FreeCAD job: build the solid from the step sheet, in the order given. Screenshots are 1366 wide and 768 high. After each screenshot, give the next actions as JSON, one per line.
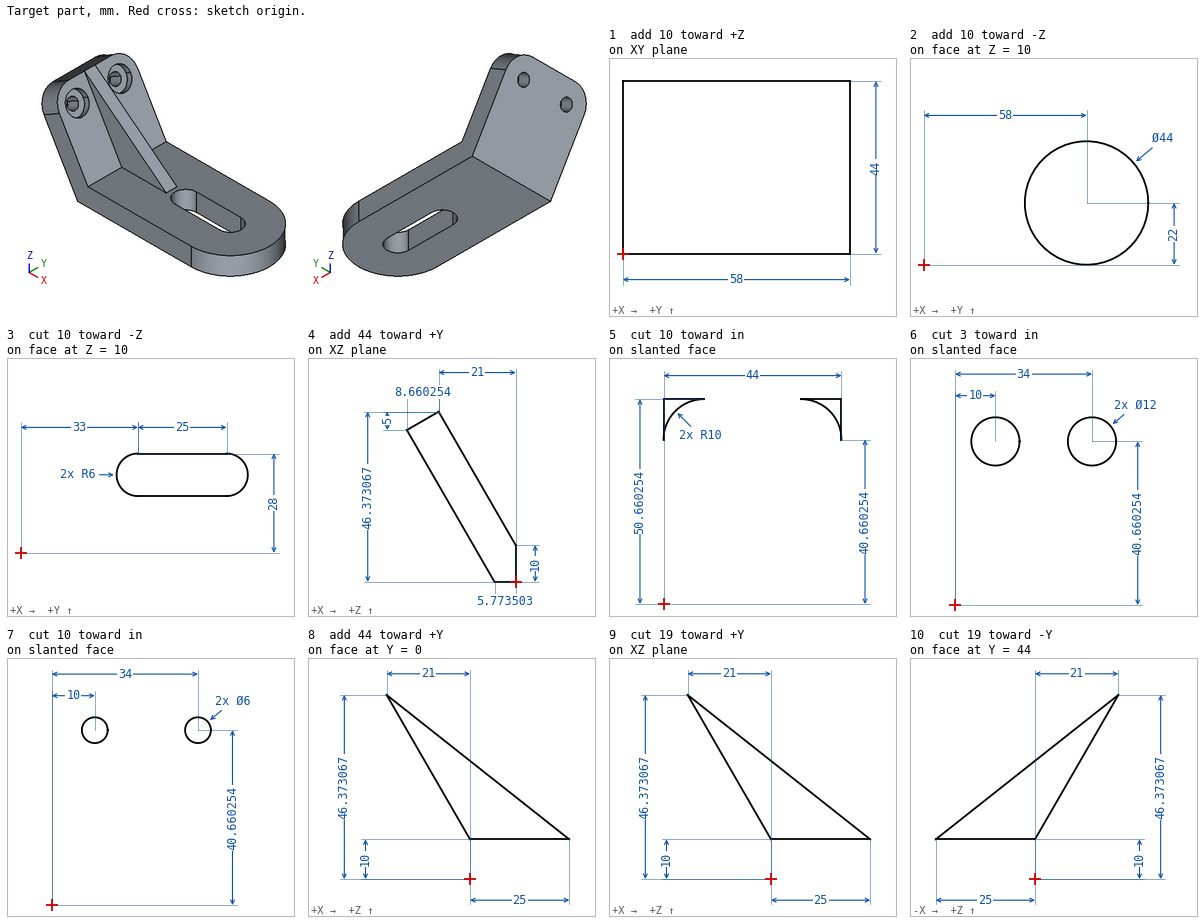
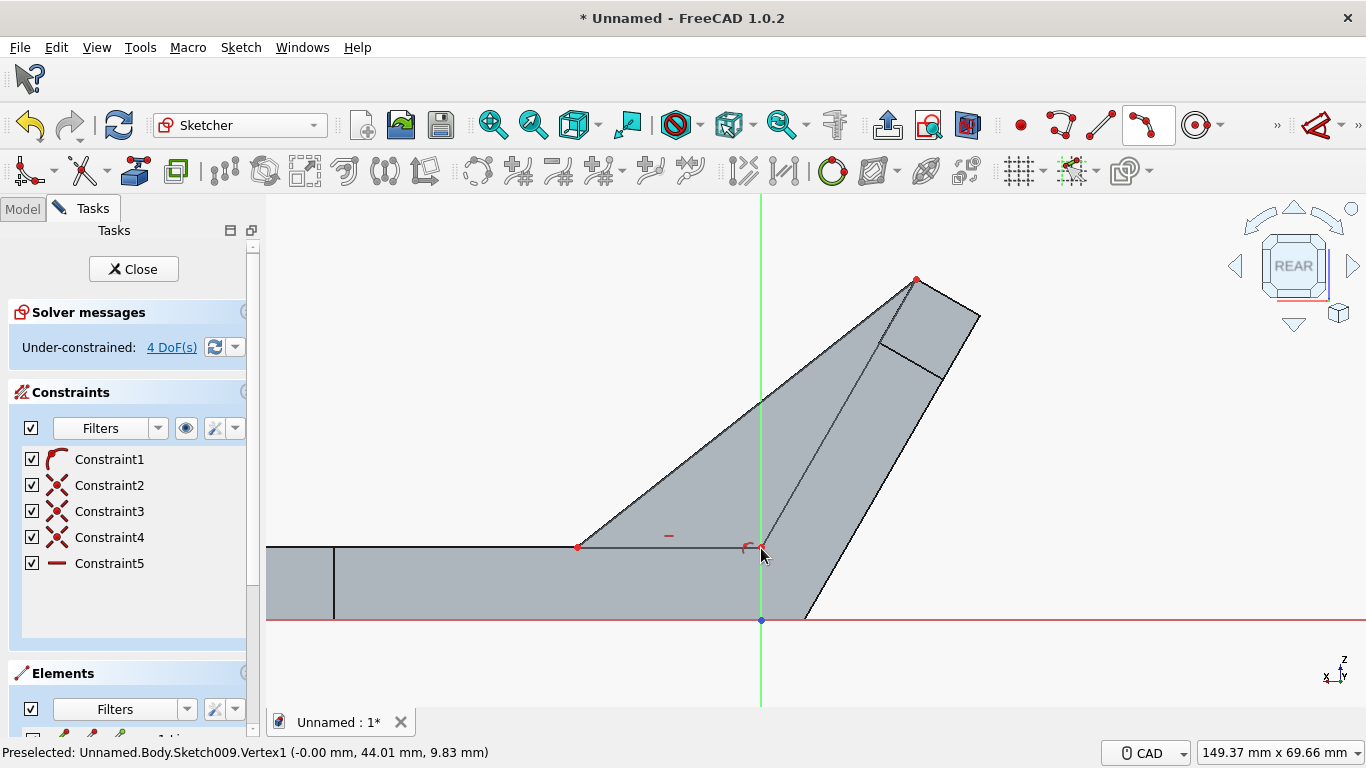
{"action": "left_click", "coordinate": [1316, 126]}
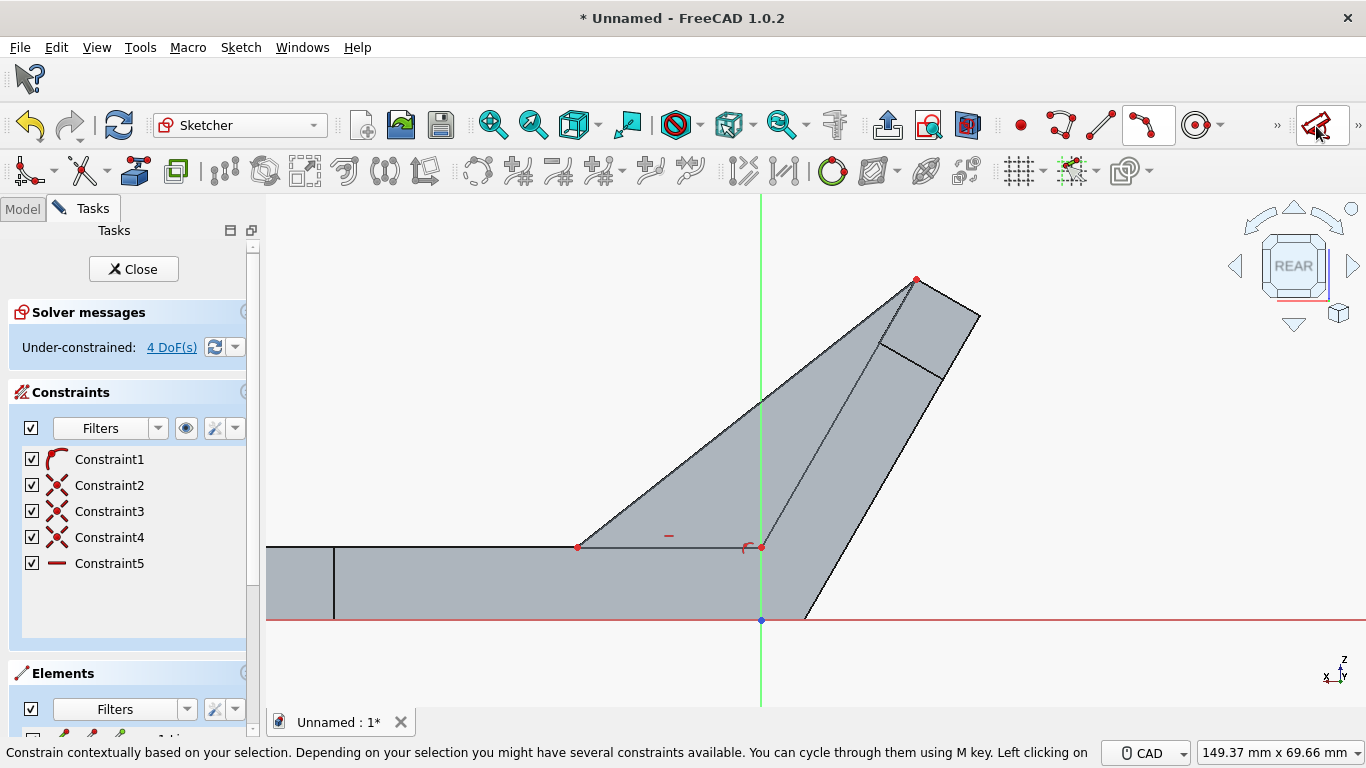
{"action": "left_click", "coordinate": [632, 548]}
{"action": "left_click", "coordinate": [669, 582]}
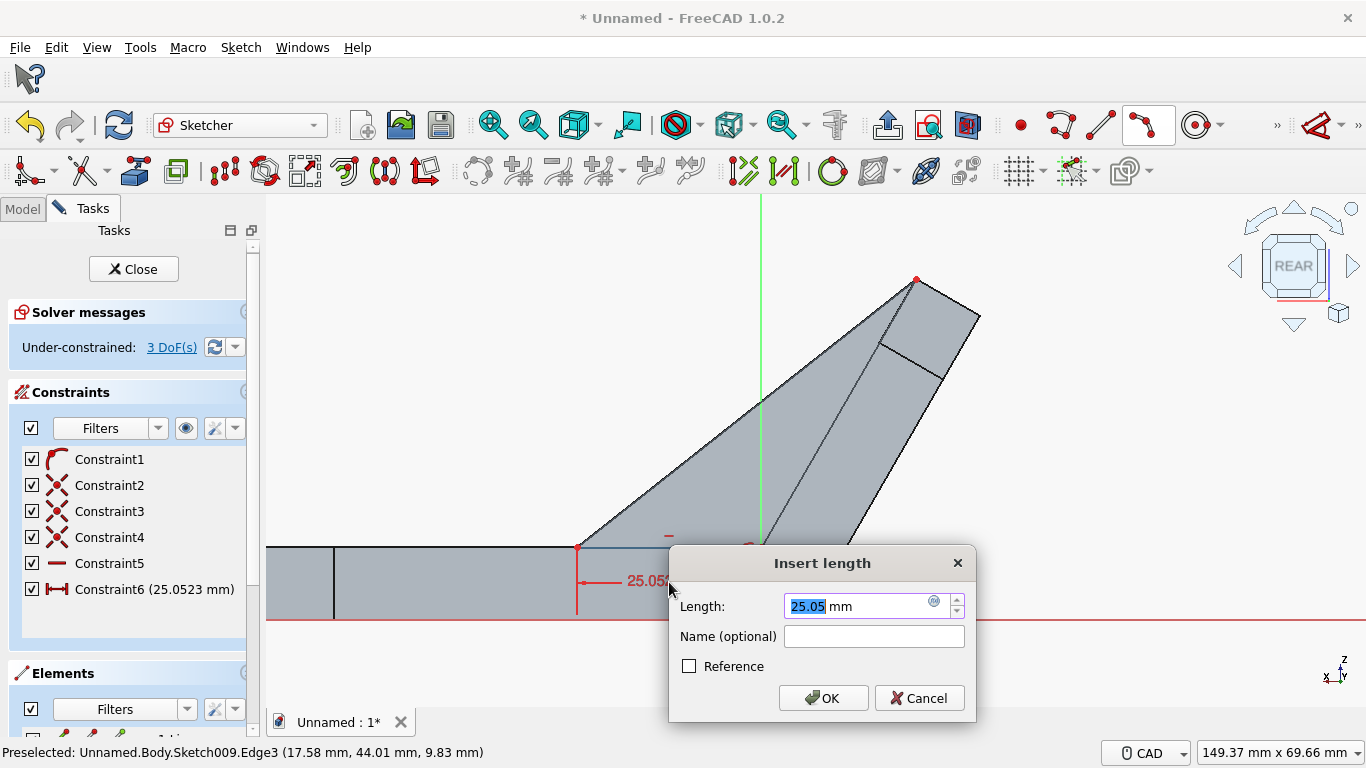
{"action": "type", "text": "25"}
{"action": "key", "text": "Return"}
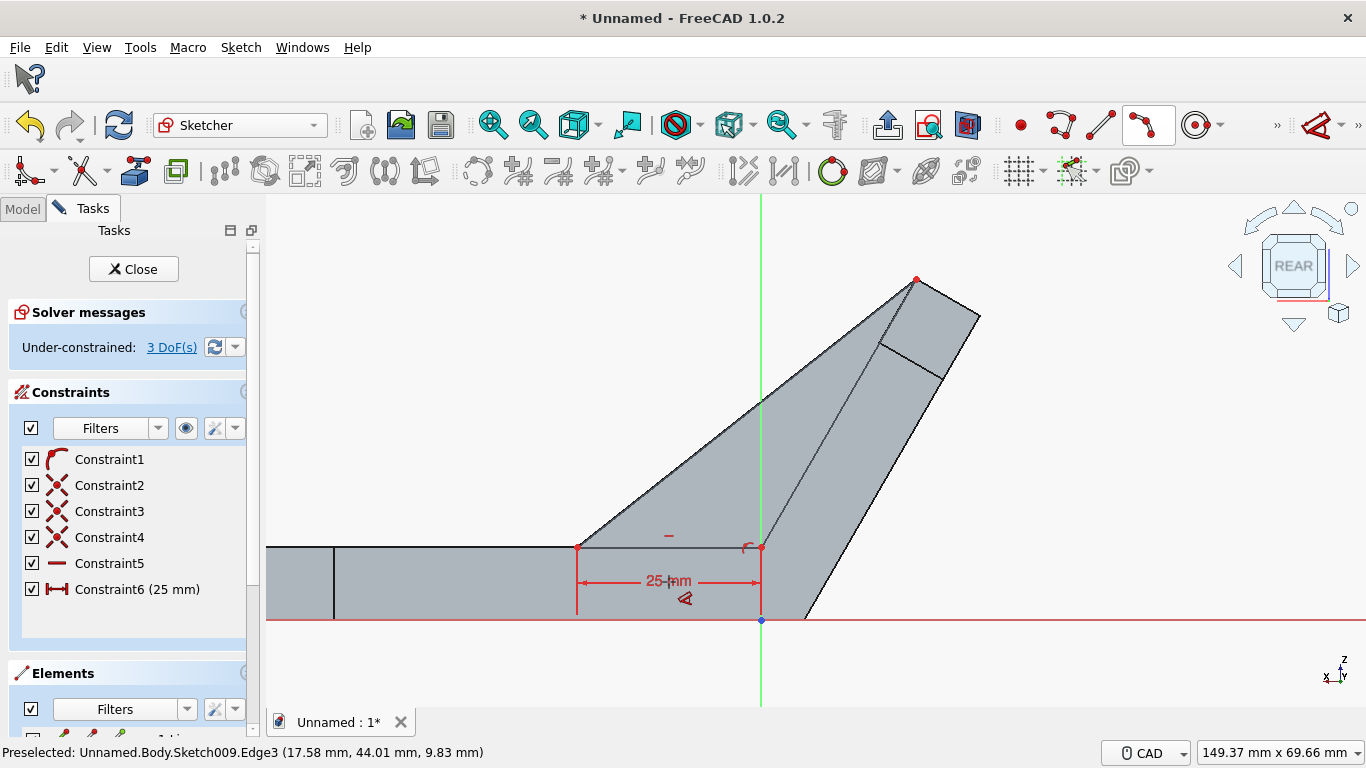
{"action": "left_click", "coordinate": [761, 548]}
{"action": "left_click", "coordinate": [795, 584]}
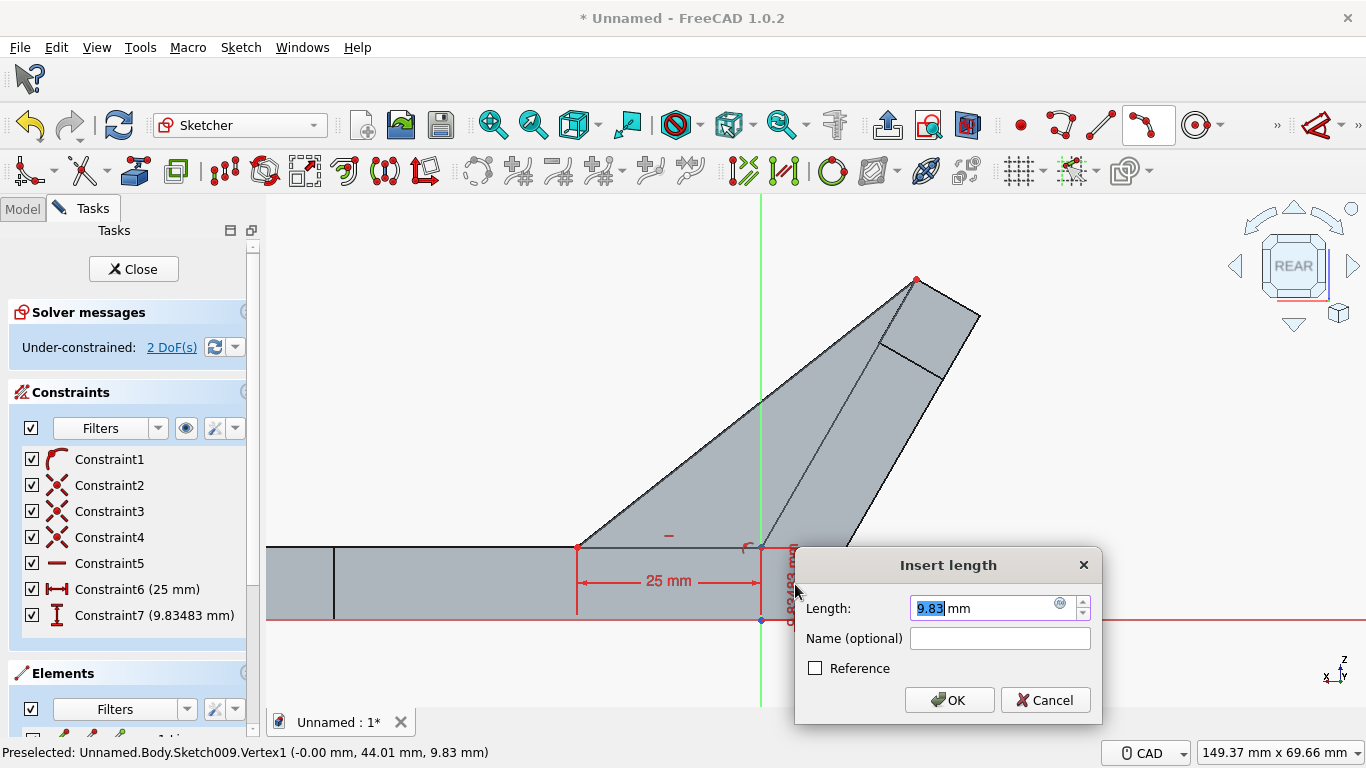
{"action": "type", "text": "10"}
{"action": "key", "text": "Return"}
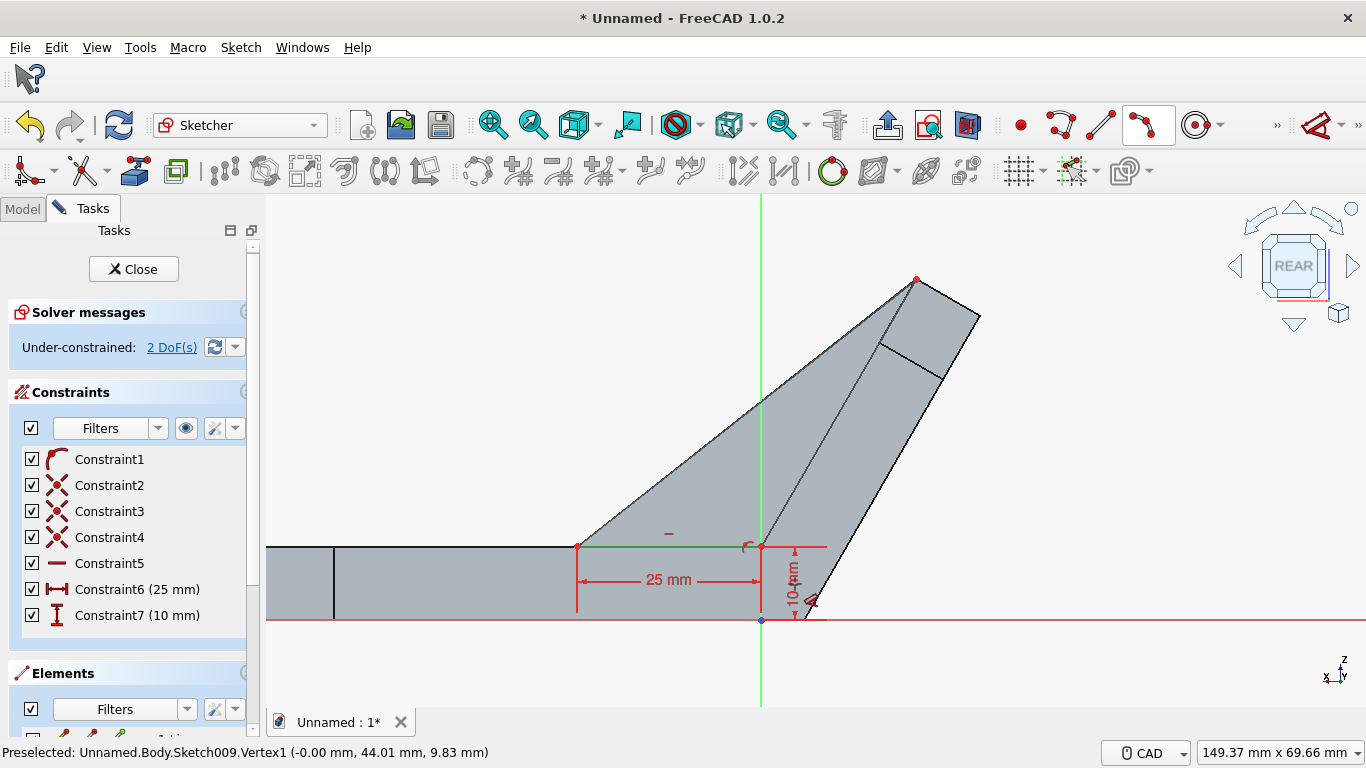
{"action": "left_click", "coordinate": [916, 280]}
{"action": "left_click", "coordinate": [839, 654]}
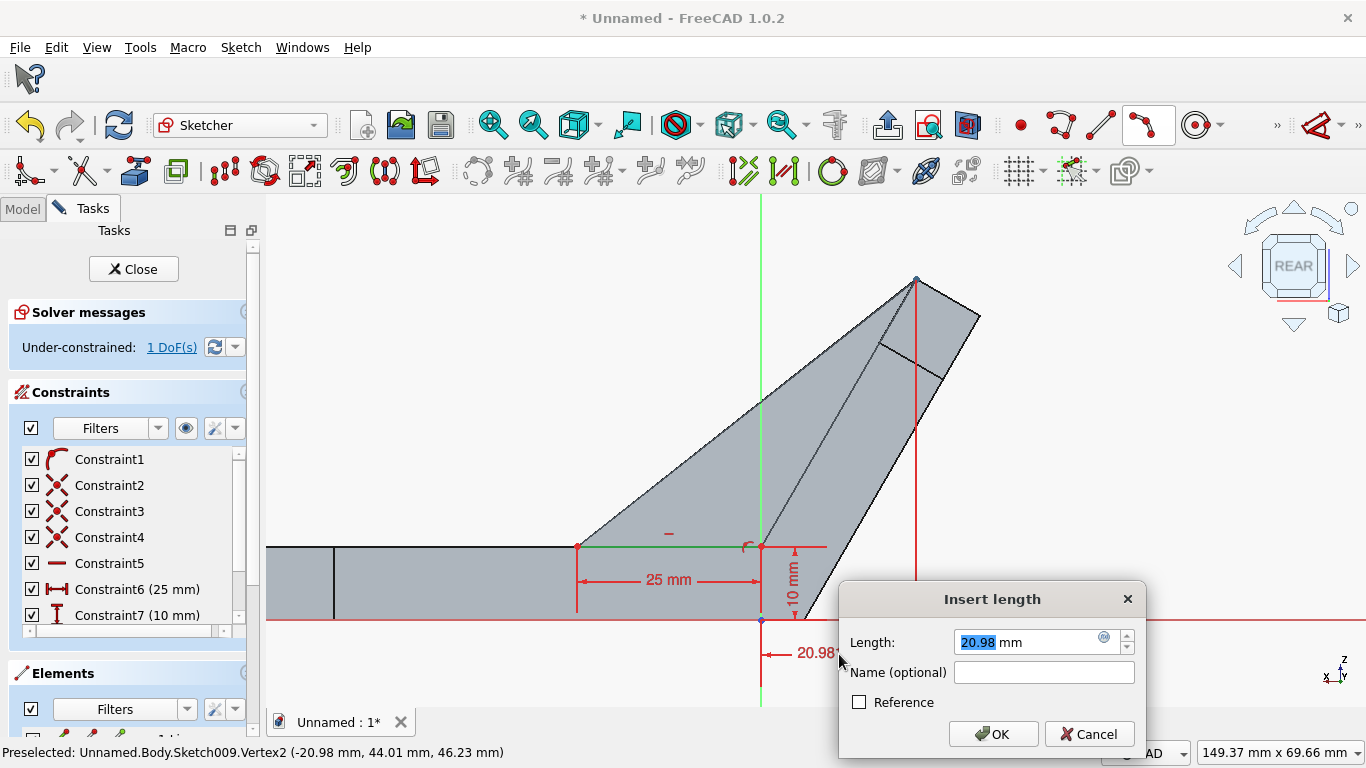
{"action": "type", "text": "21"}
{"action": "key", "text": "Return"}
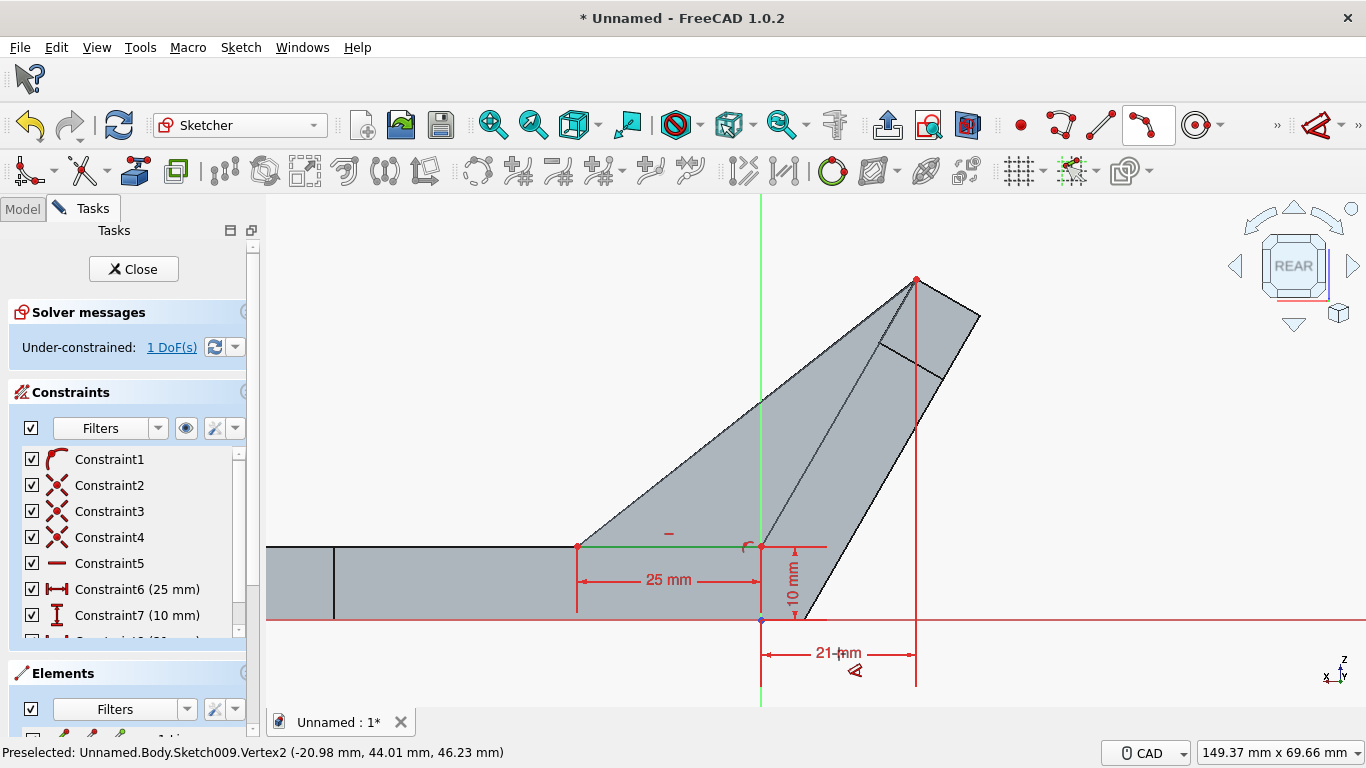
{"action": "left_click", "coordinate": [916, 280]}
{"action": "left_click", "coordinate": [950, 450]}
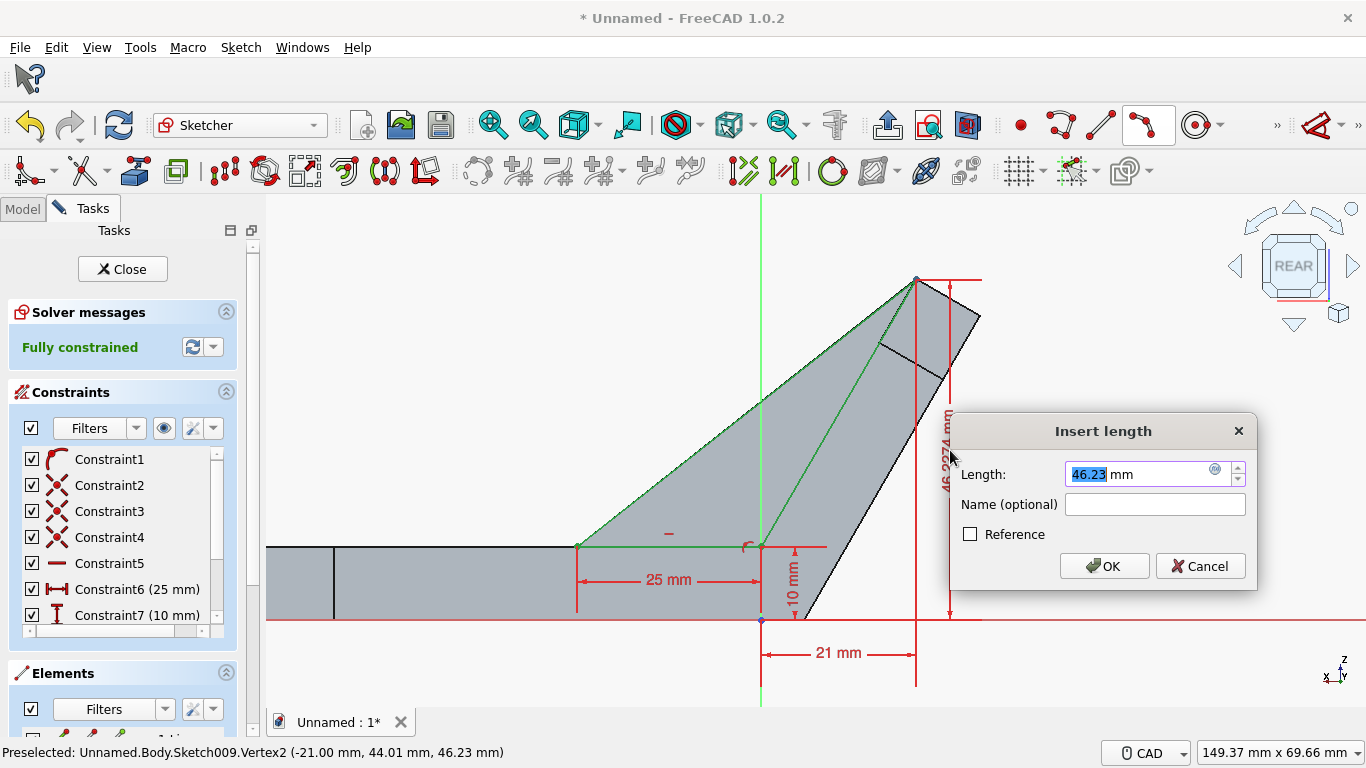
{"action": "type", "text": "46.373067"}
{"action": "key", "text": "Return"}
{"action": "key", "text": "Escape"}